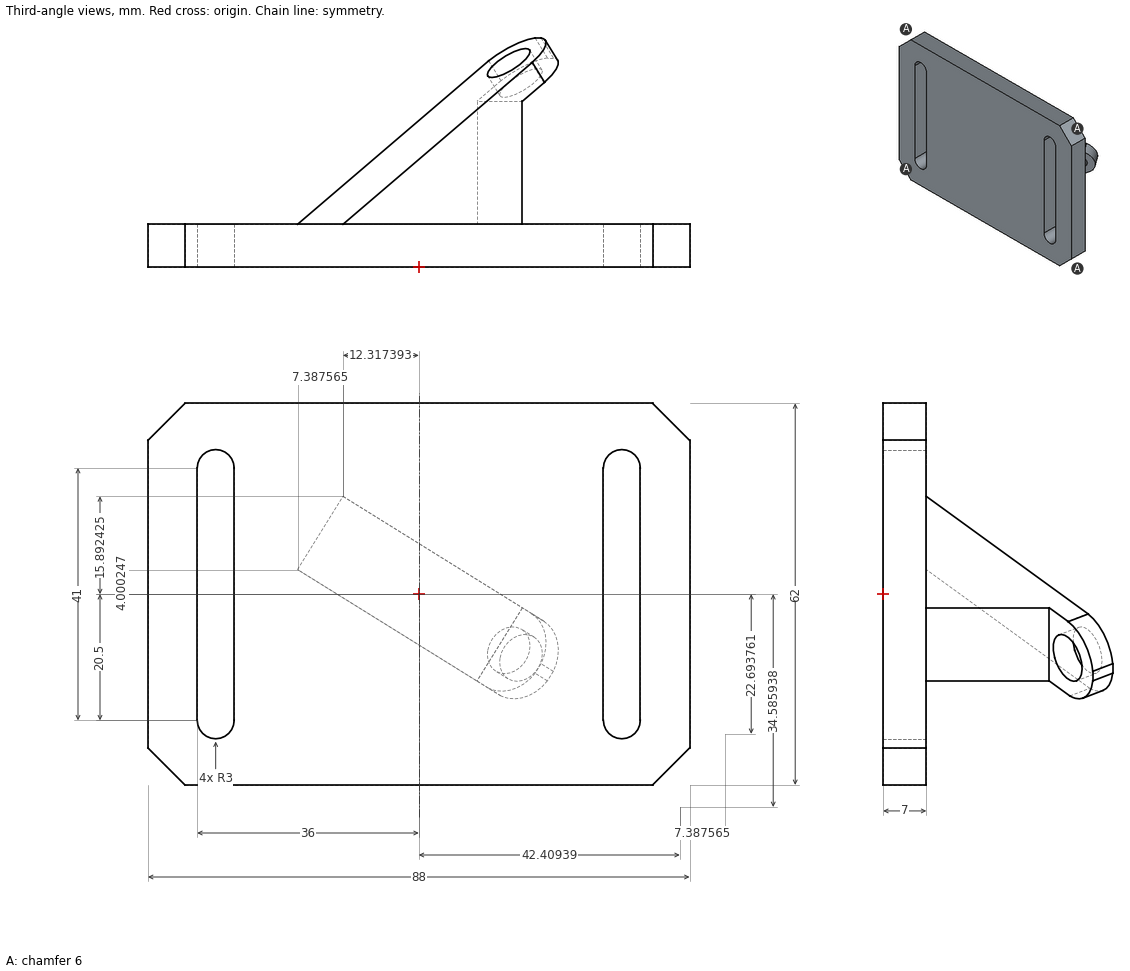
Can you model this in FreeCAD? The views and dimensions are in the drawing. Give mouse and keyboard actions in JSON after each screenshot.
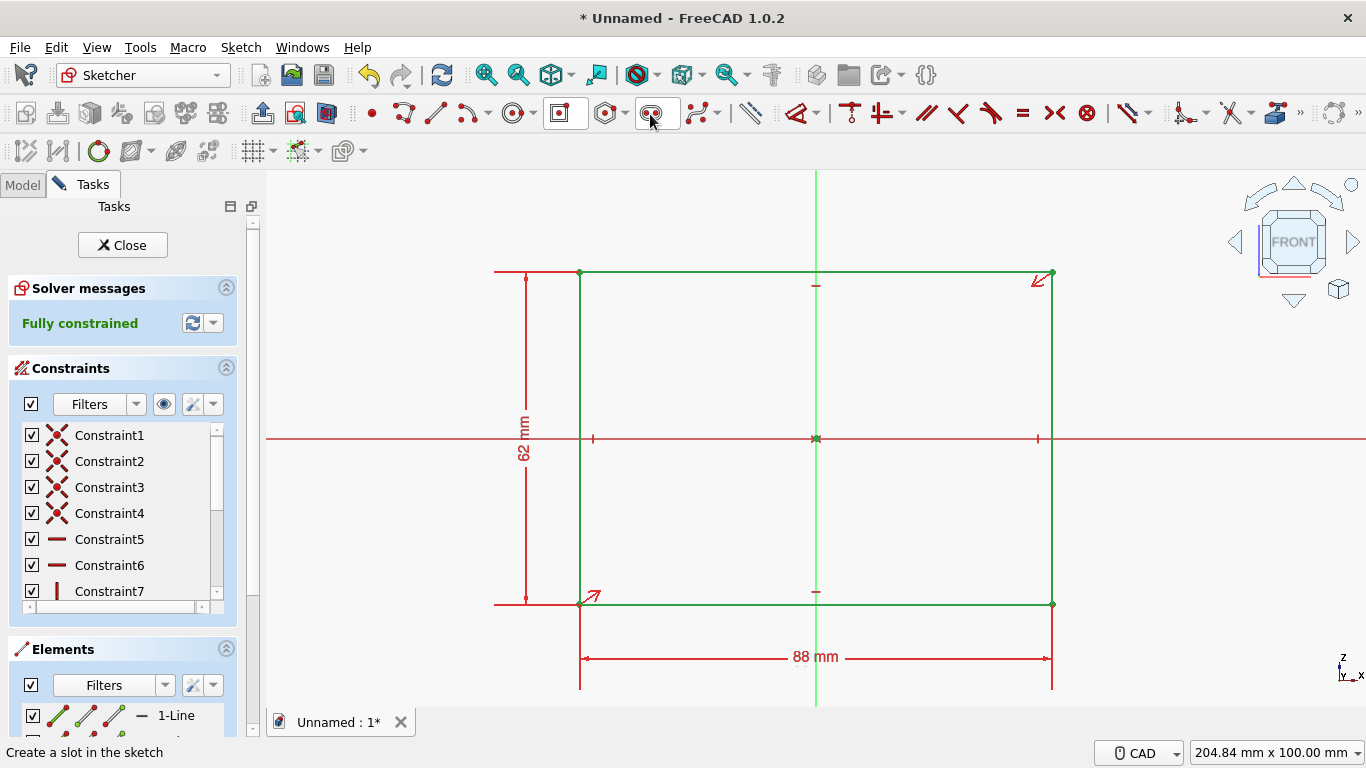
{"action": "scroll", "coordinate": [639, 549], "scroll_direction": "up", "scroll_amount": 2}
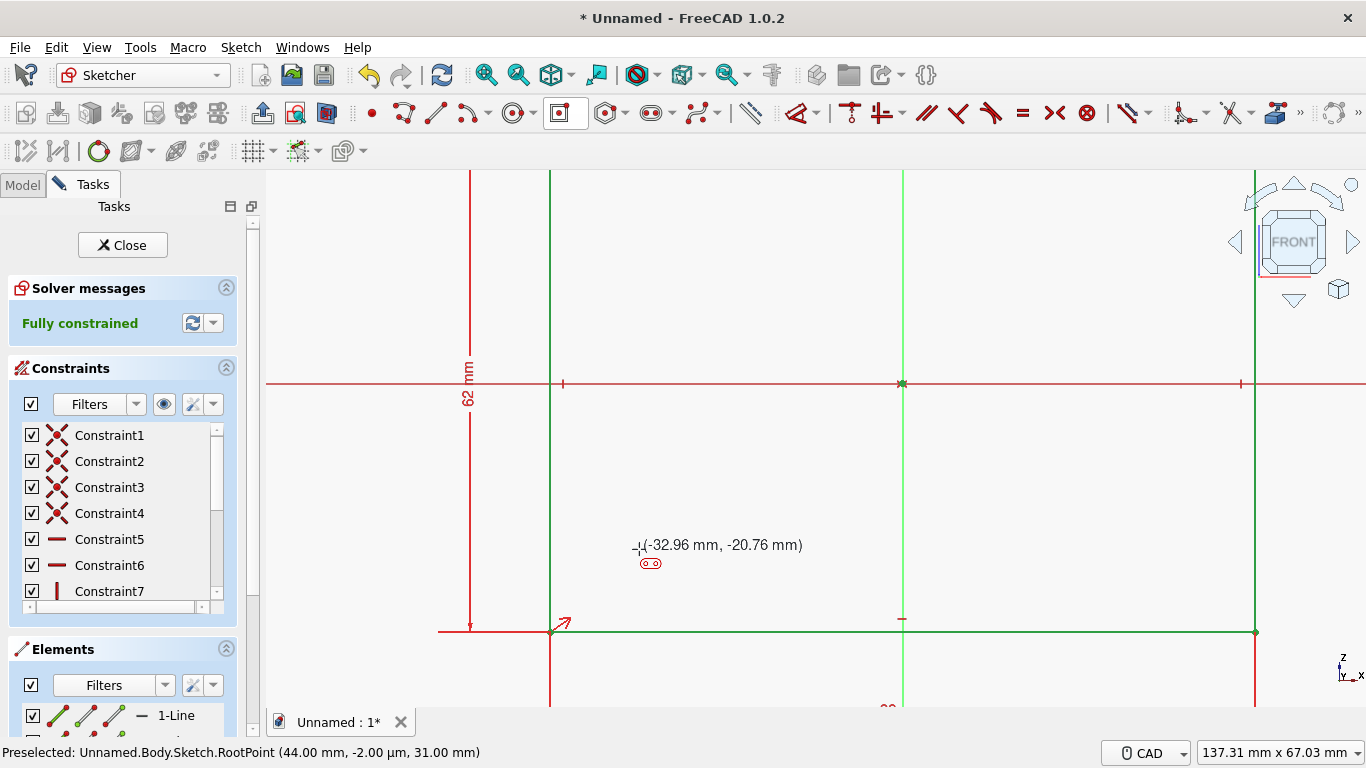
{"action": "left_click", "coordinate": [639, 548]}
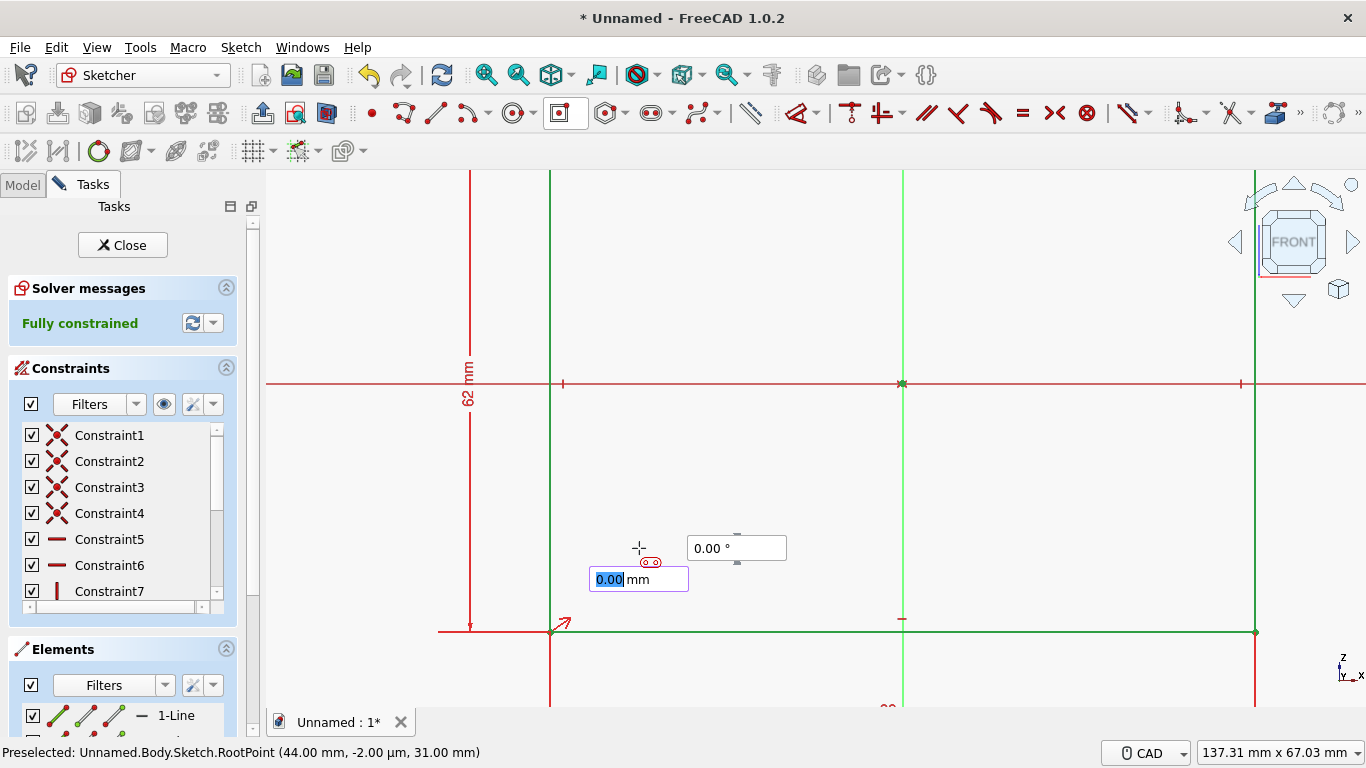
{"action": "left_click", "coordinate": [639, 220]}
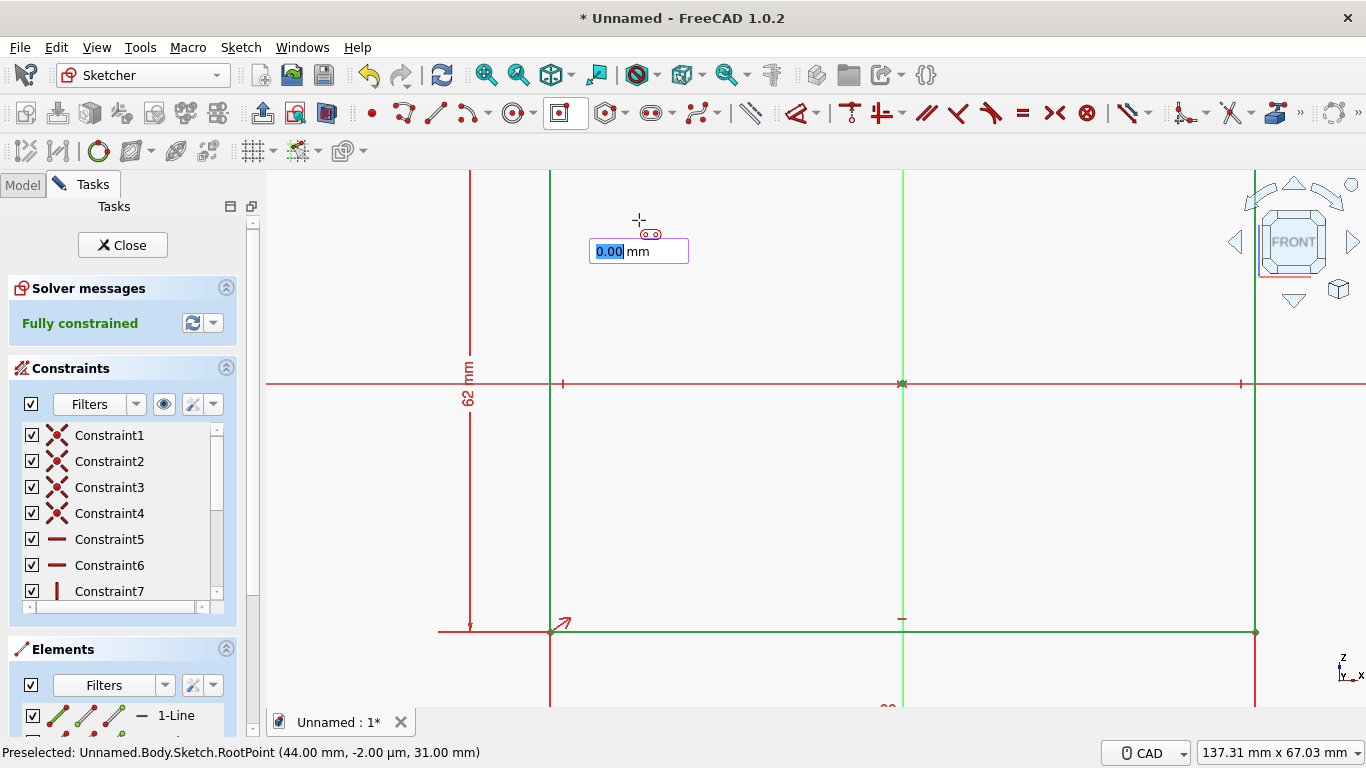
{"action": "left_click", "coordinate": [663, 433]}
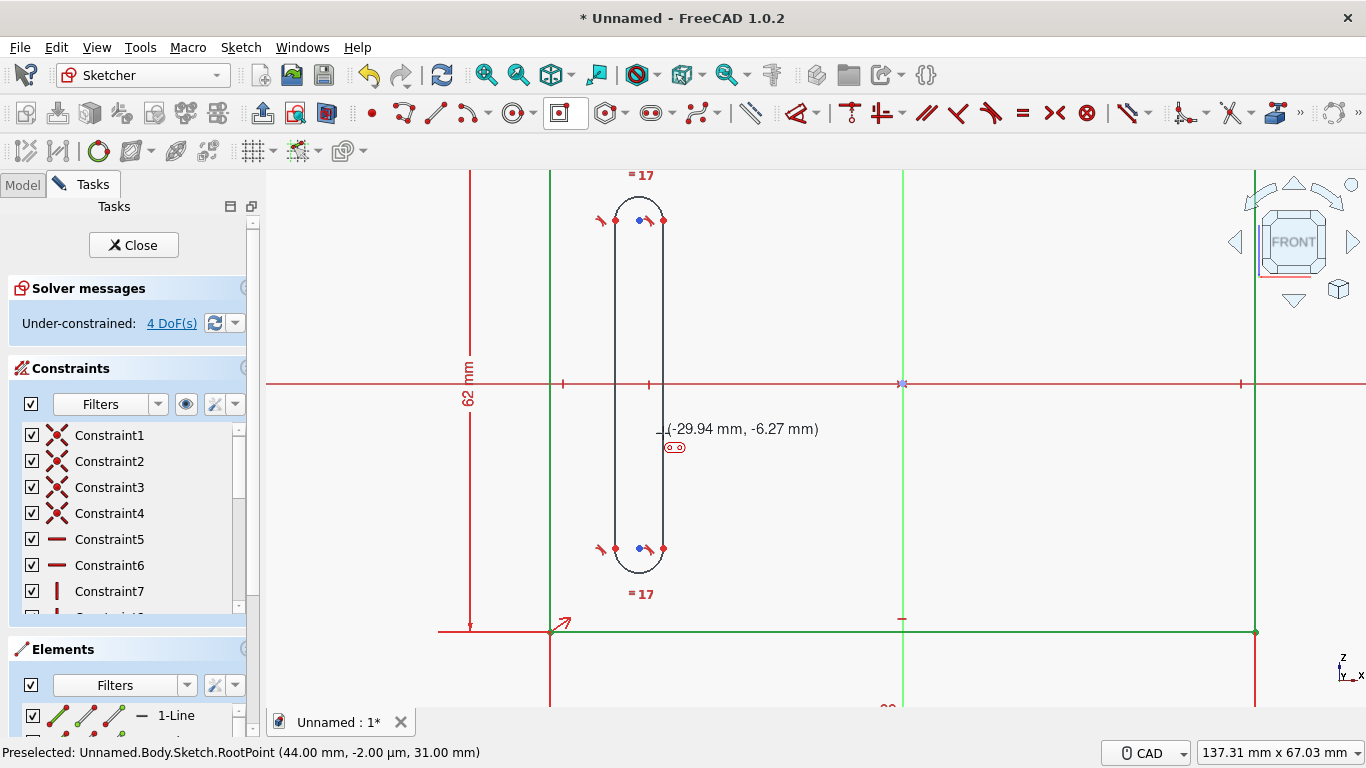
{"action": "left_click", "coordinate": [1167, 548]}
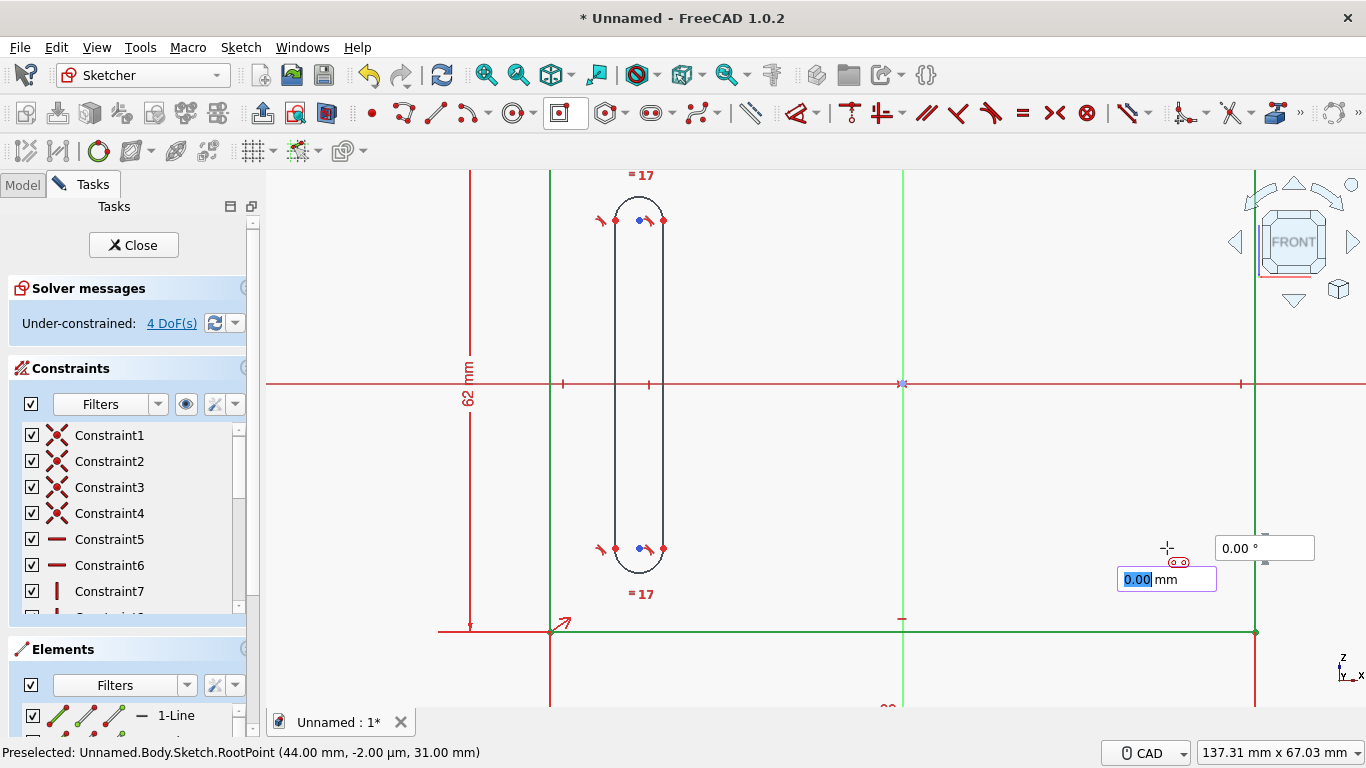
{"action": "left_click", "coordinate": [1167, 220]}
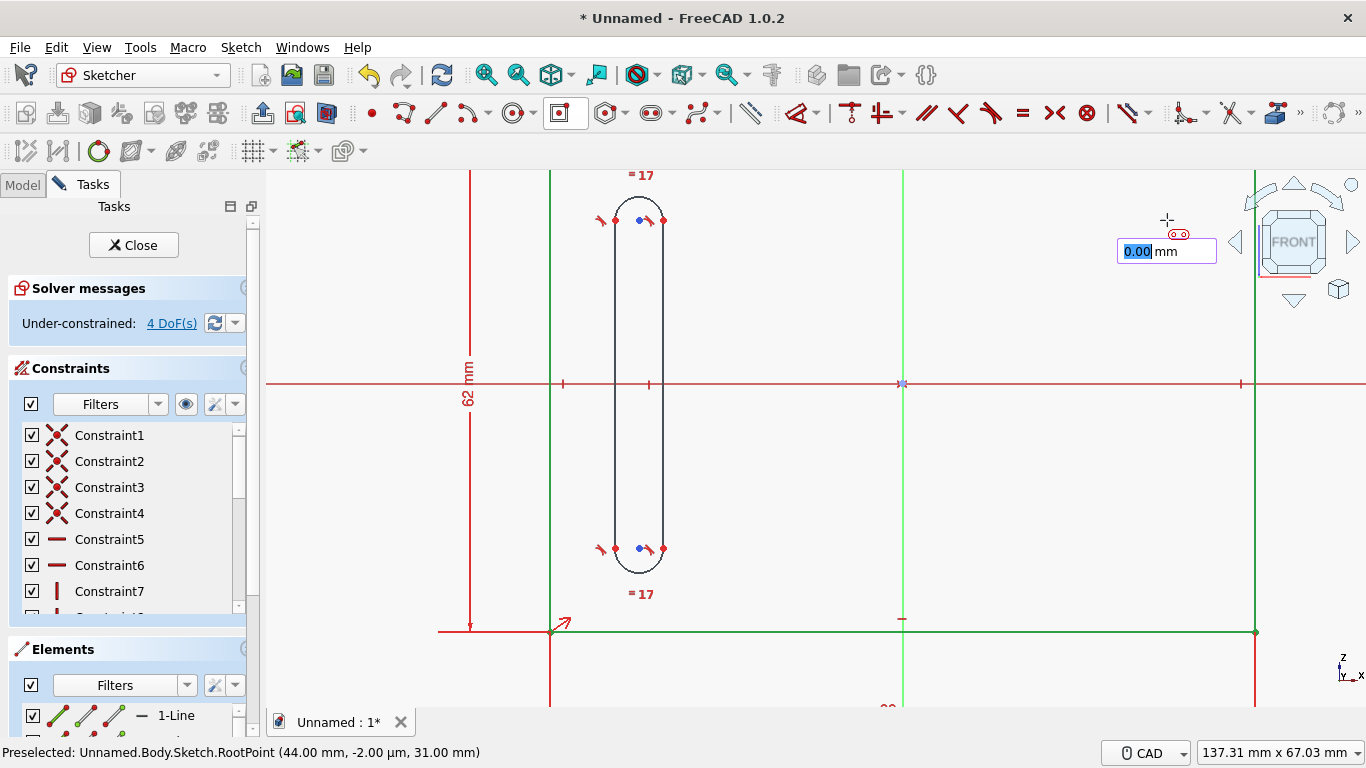
{"action": "left_click", "coordinate": [1191, 433]}
{"action": "key", "text": "Escape"}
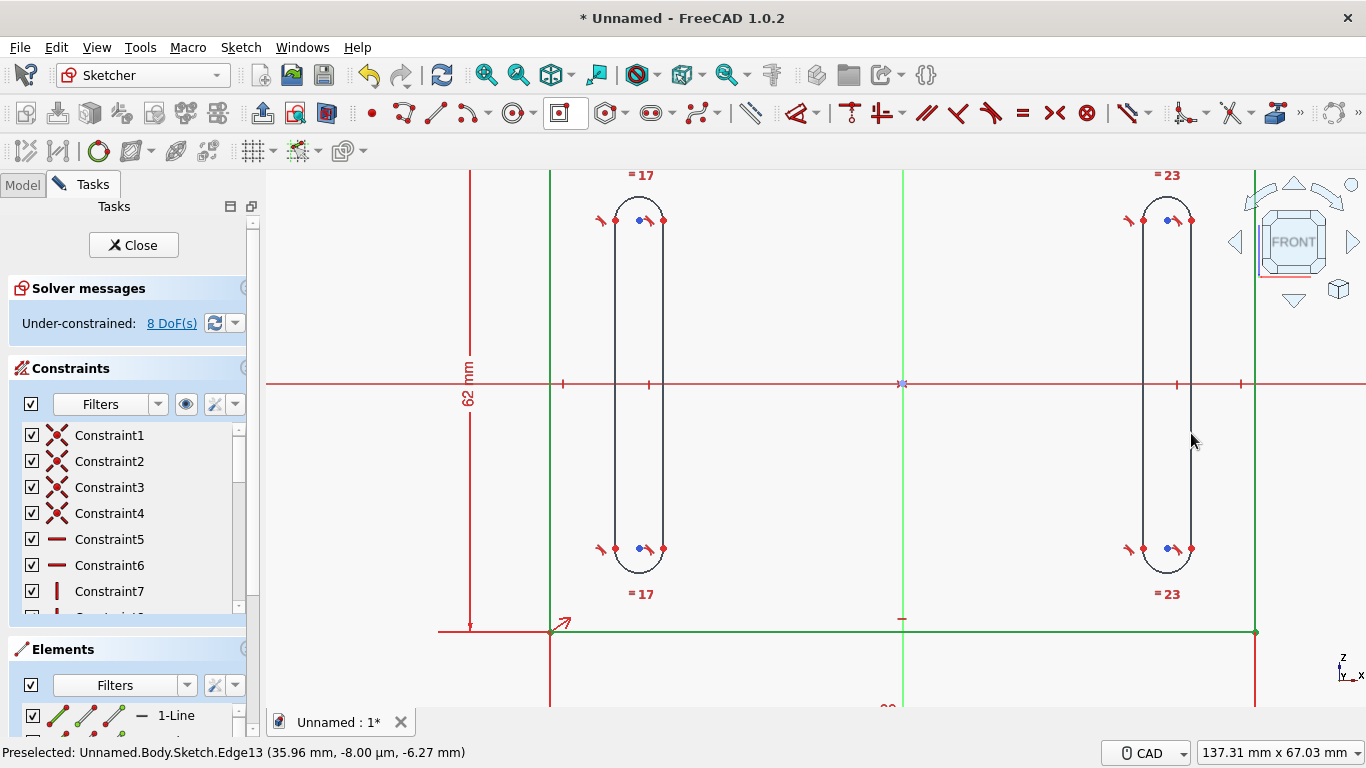
{"action": "left_click", "coordinate": [625, 568]}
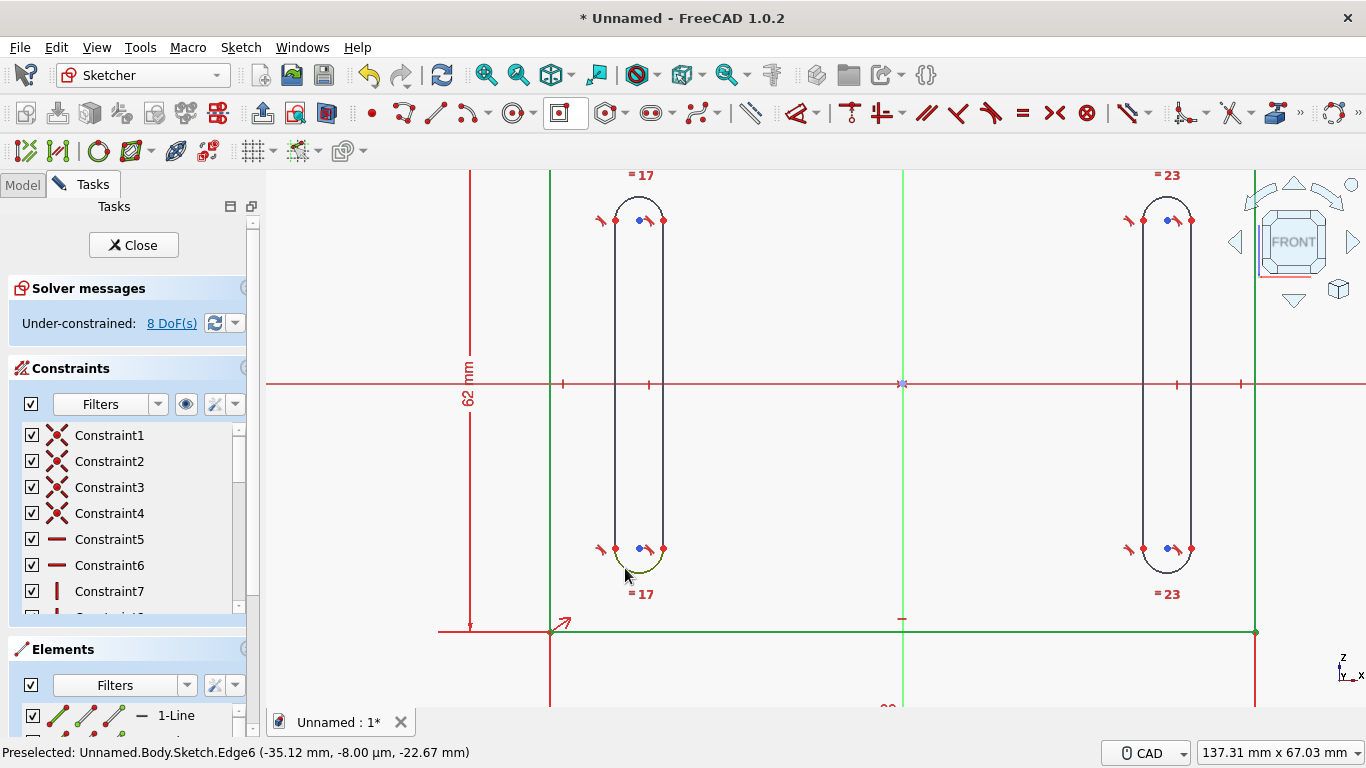
{"action": "left_click", "coordinate": [1153, 568]}